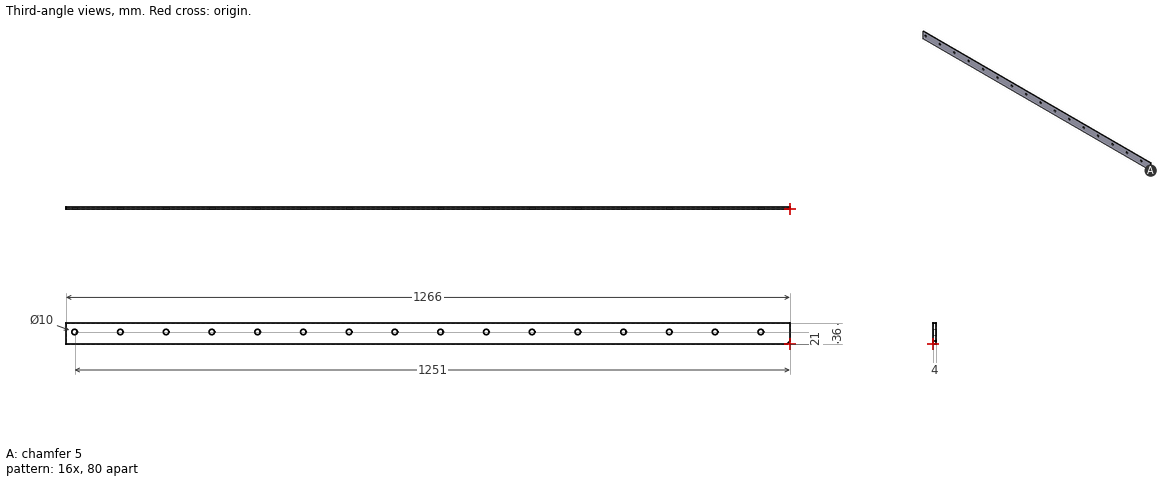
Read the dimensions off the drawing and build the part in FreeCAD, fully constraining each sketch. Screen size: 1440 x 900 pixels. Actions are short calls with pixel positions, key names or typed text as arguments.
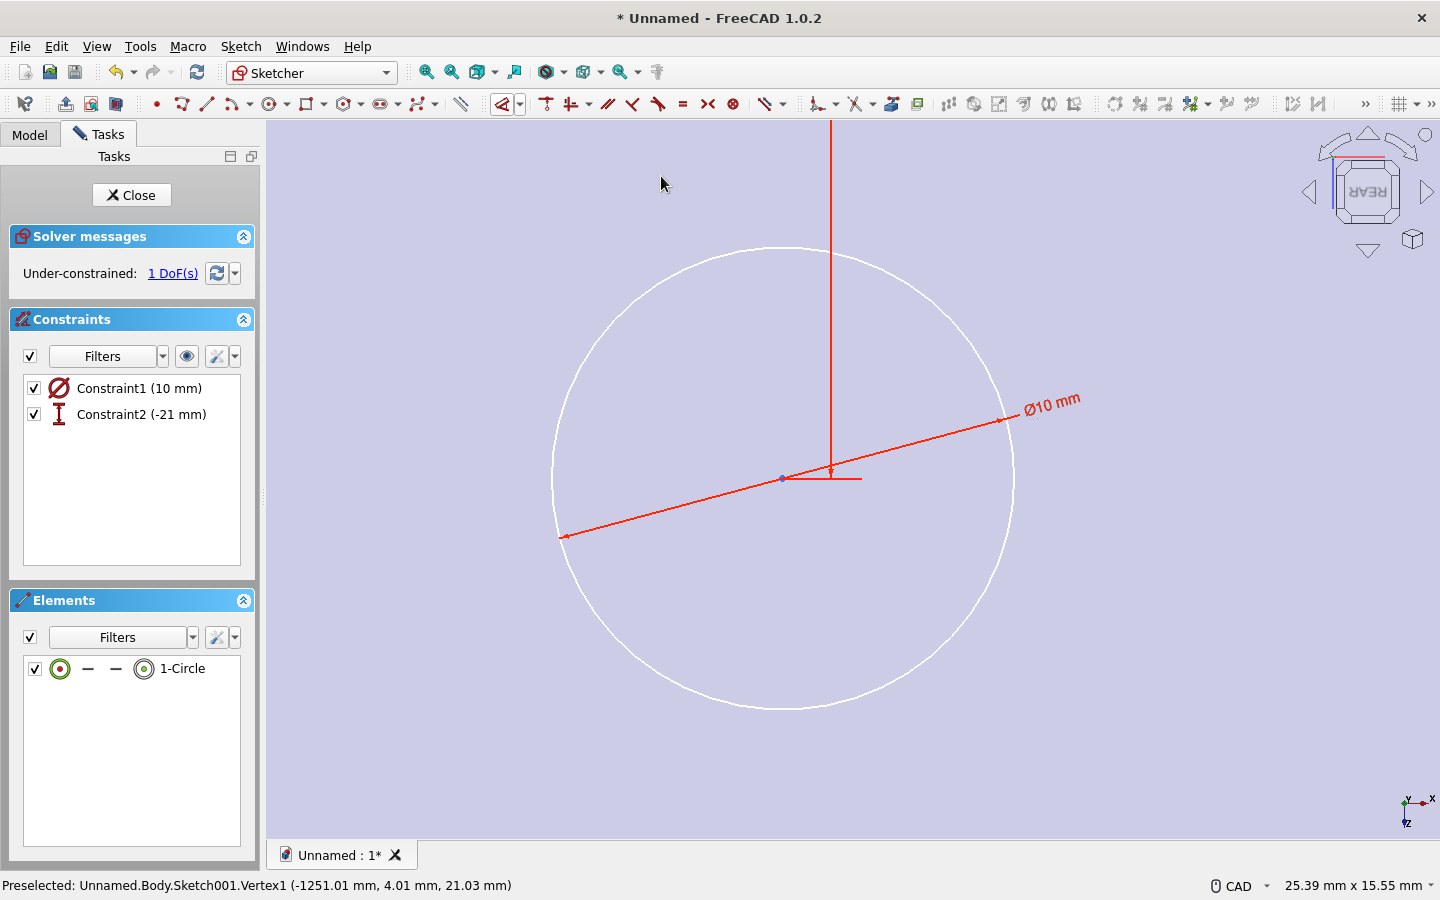
click(783, 479)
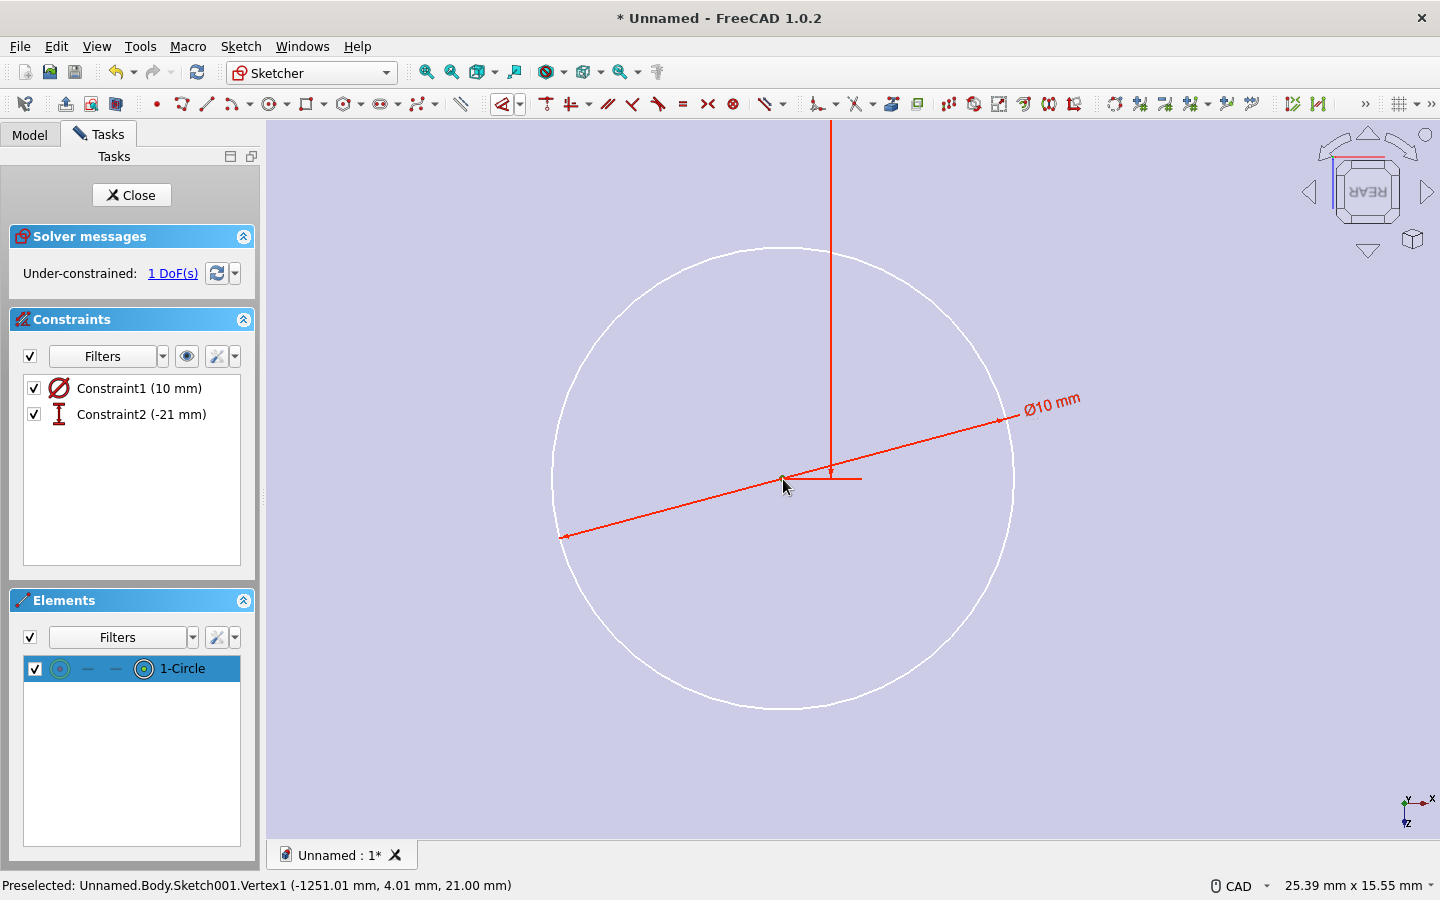
click(520, 104)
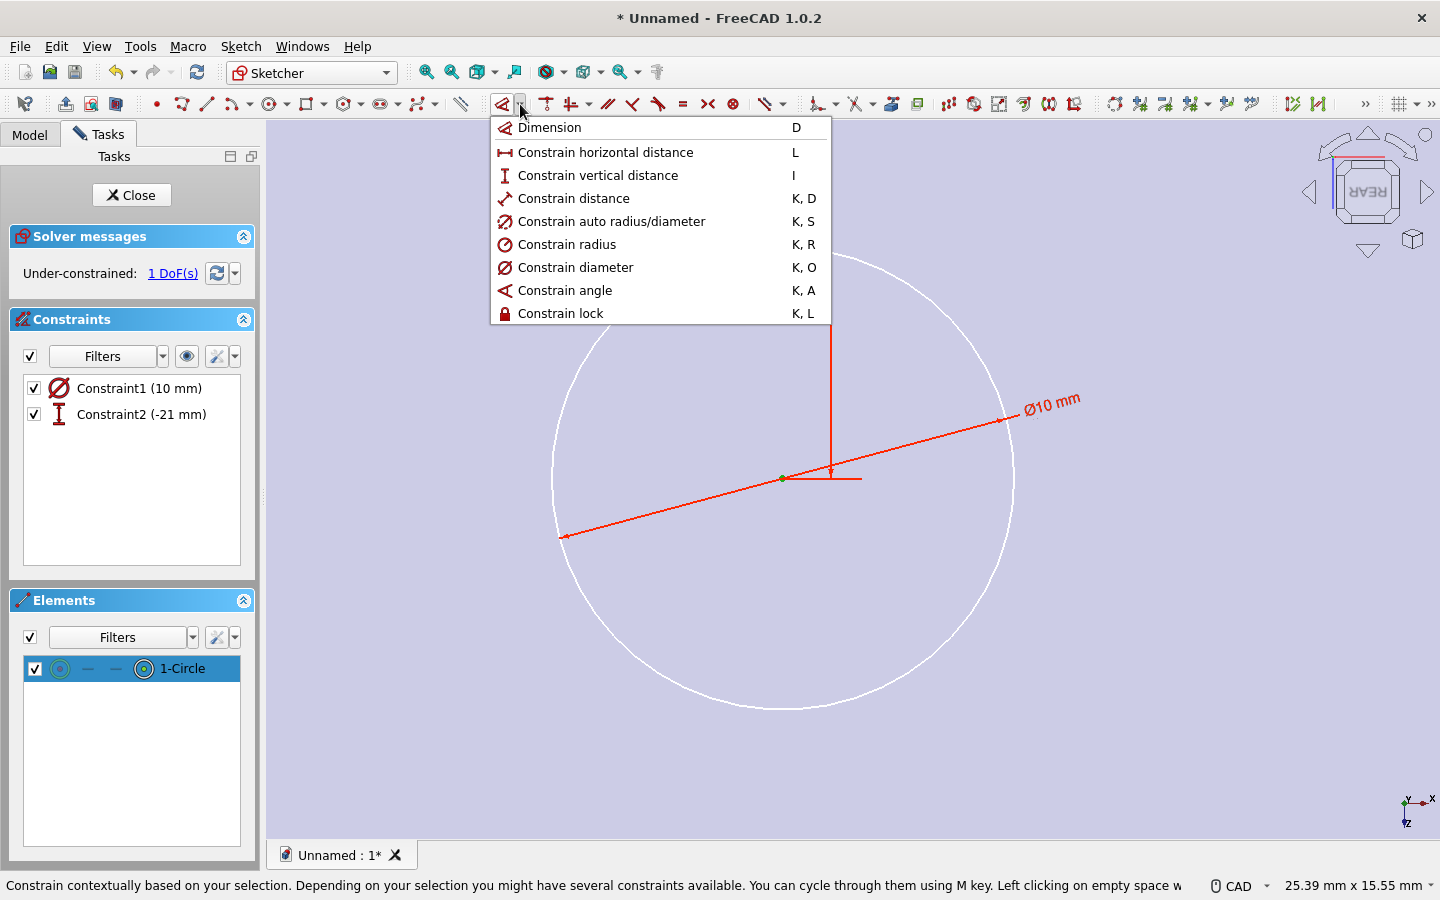
click(661, 152)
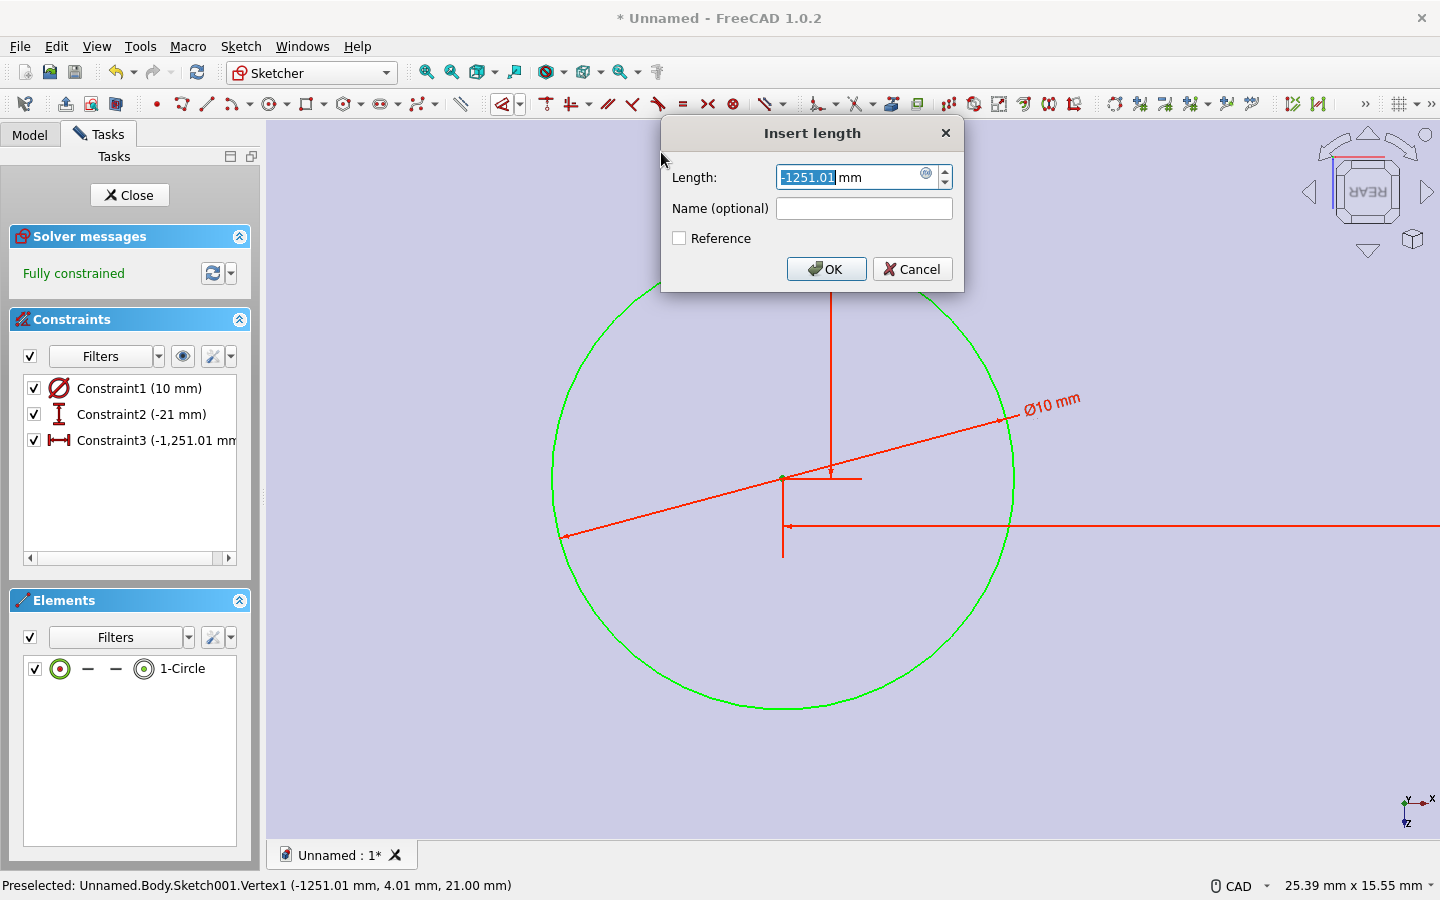
text(-1251)
key(Return)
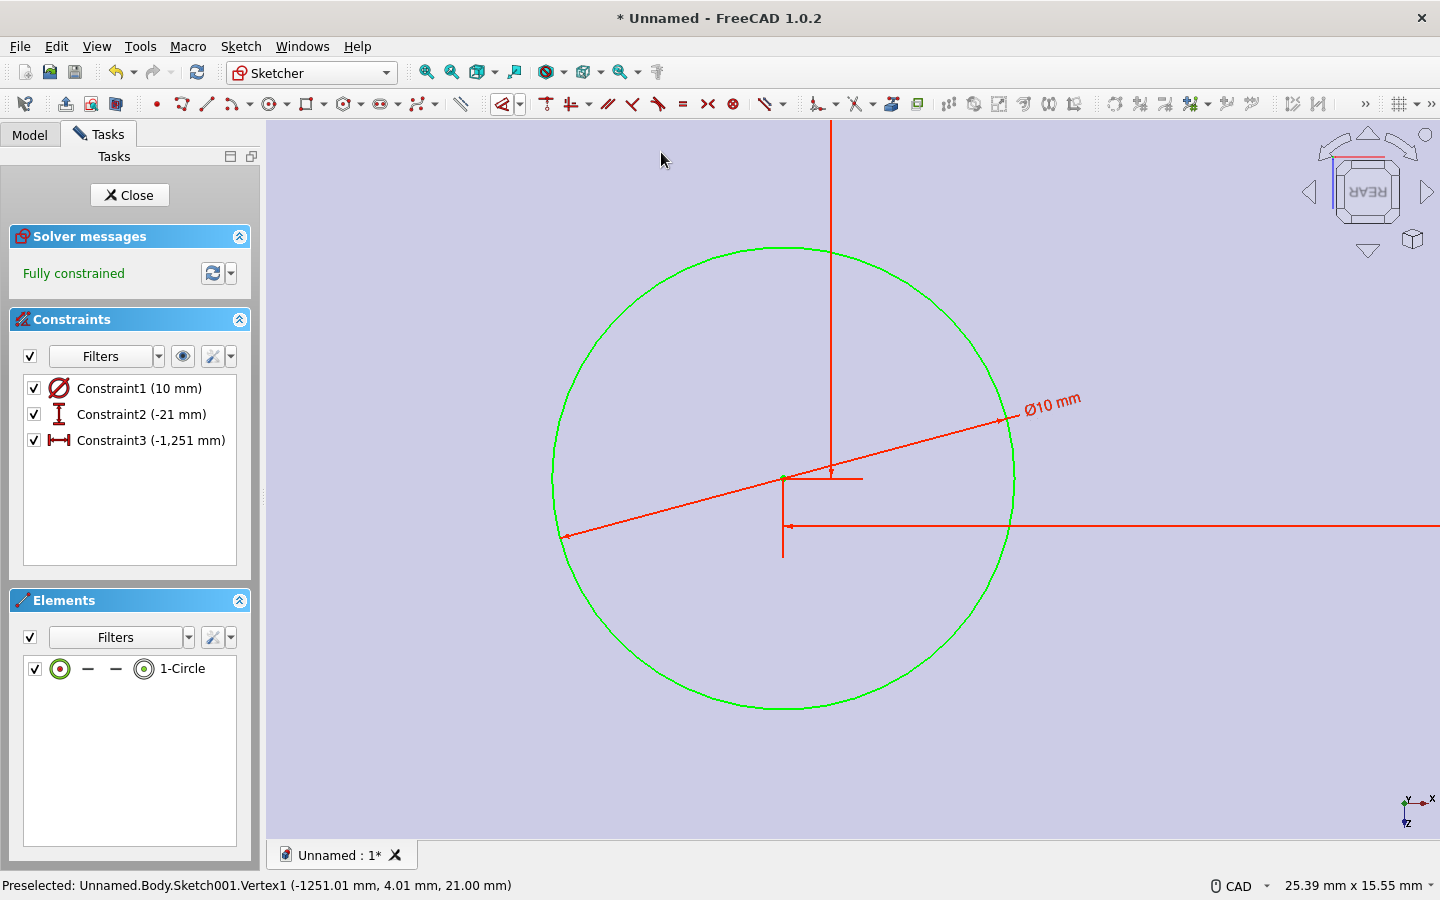
click(130, 195)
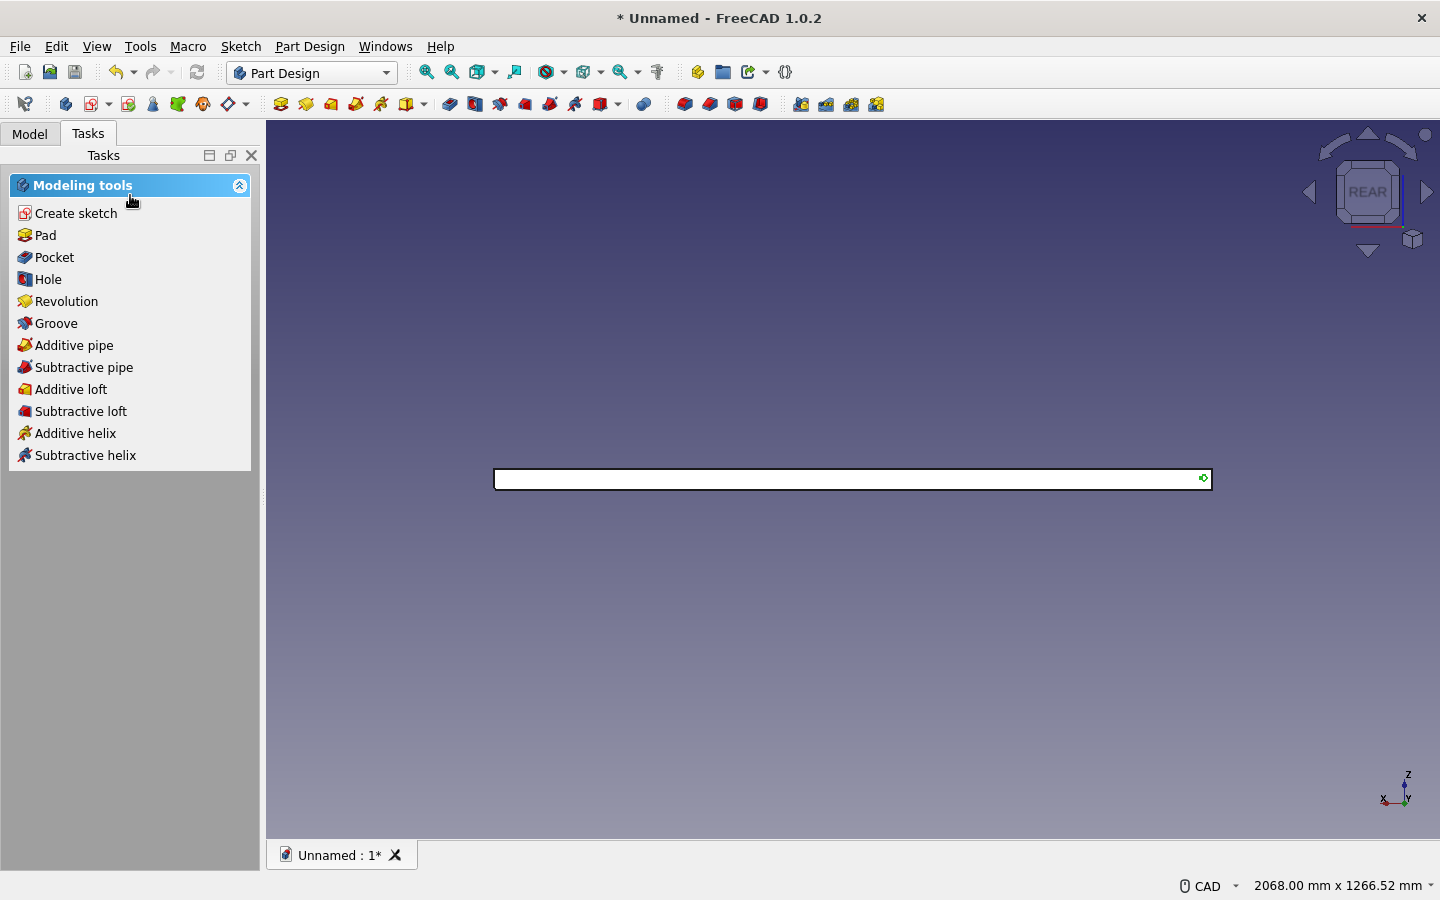
click(450, 104)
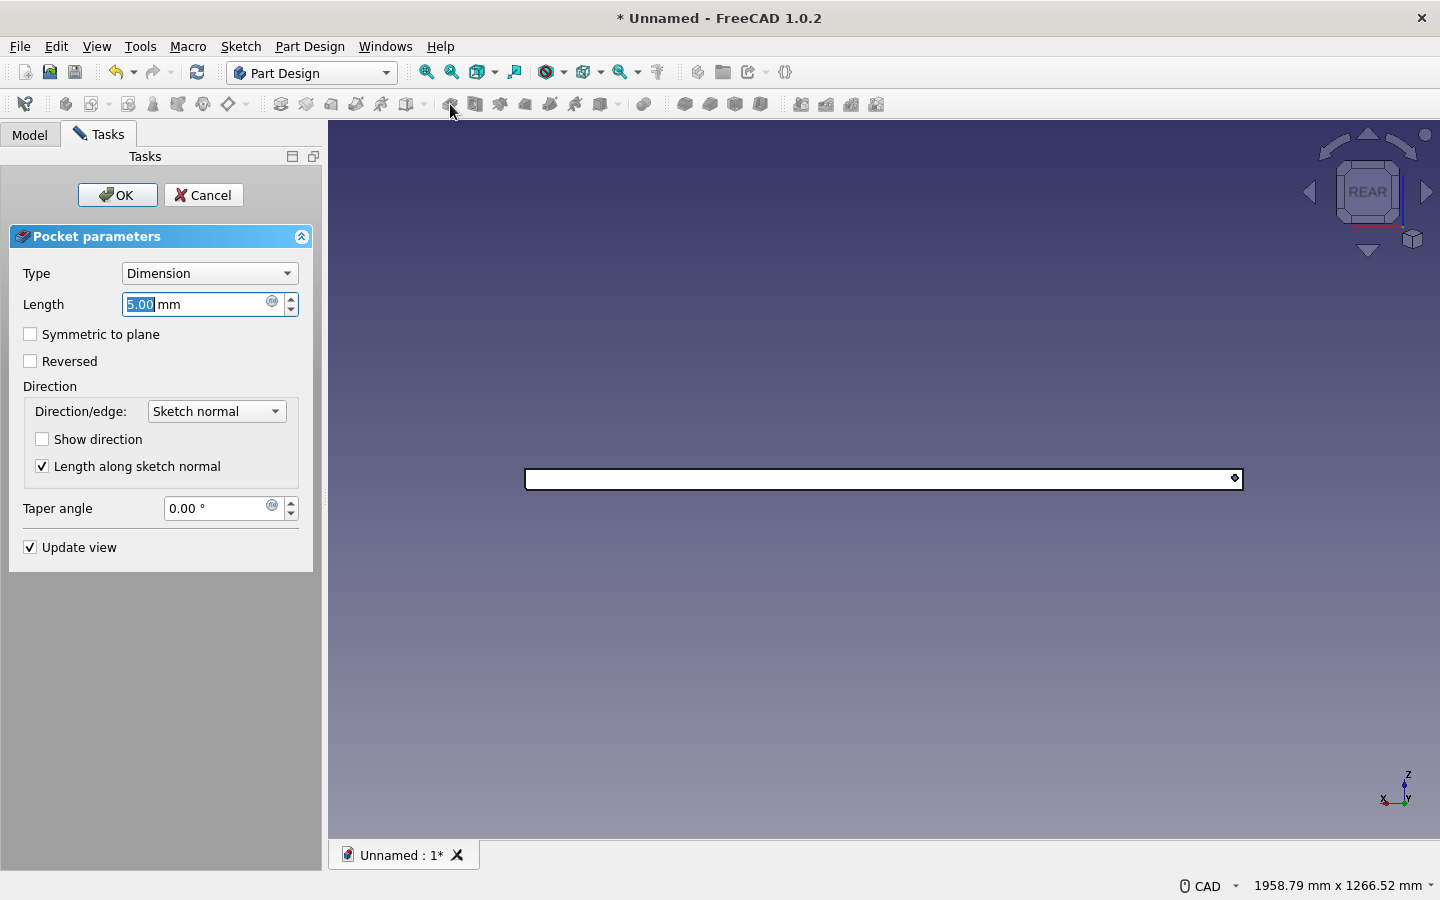
click(210, 274)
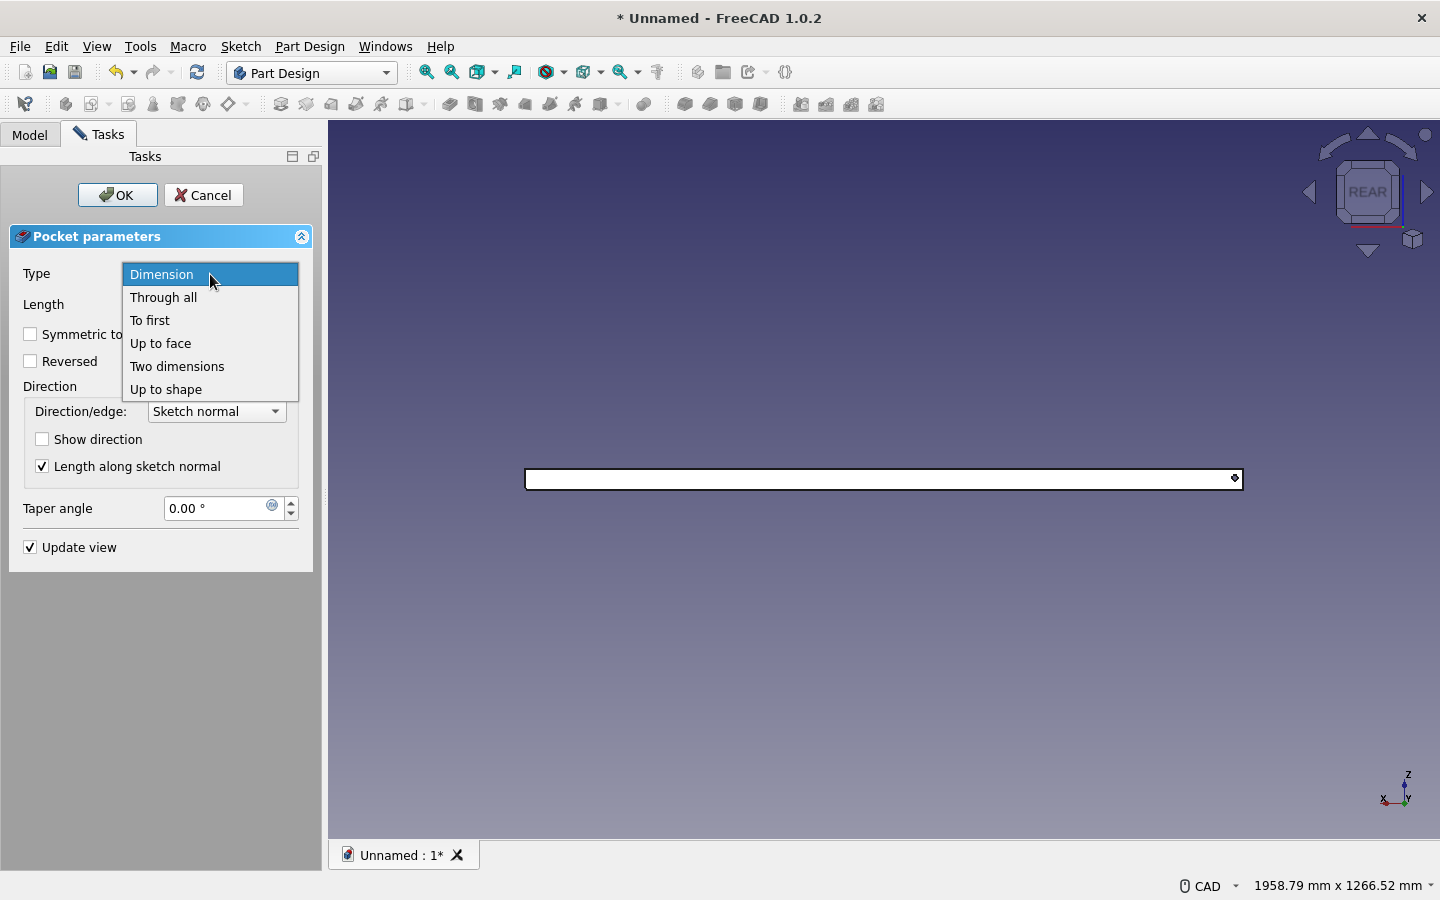
click(208, 298)